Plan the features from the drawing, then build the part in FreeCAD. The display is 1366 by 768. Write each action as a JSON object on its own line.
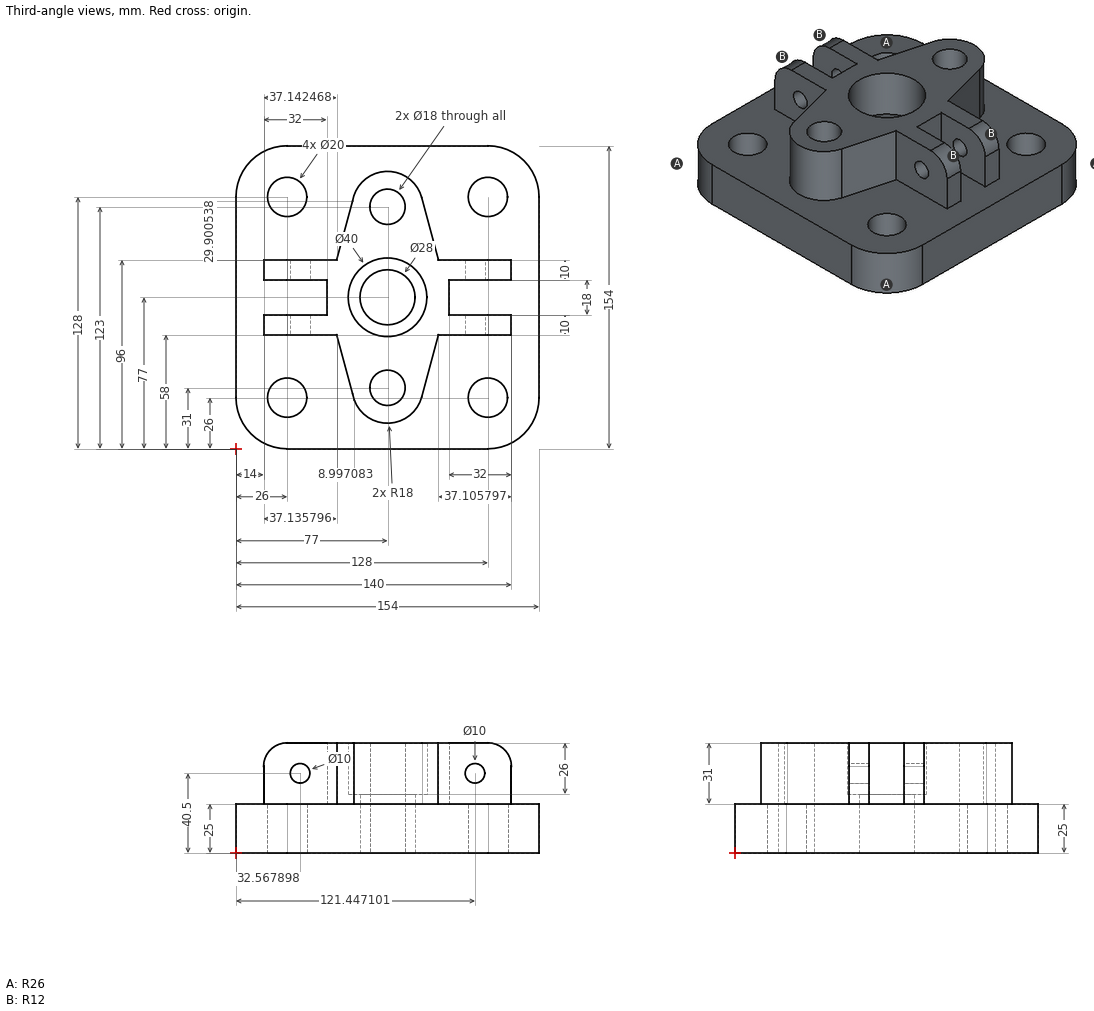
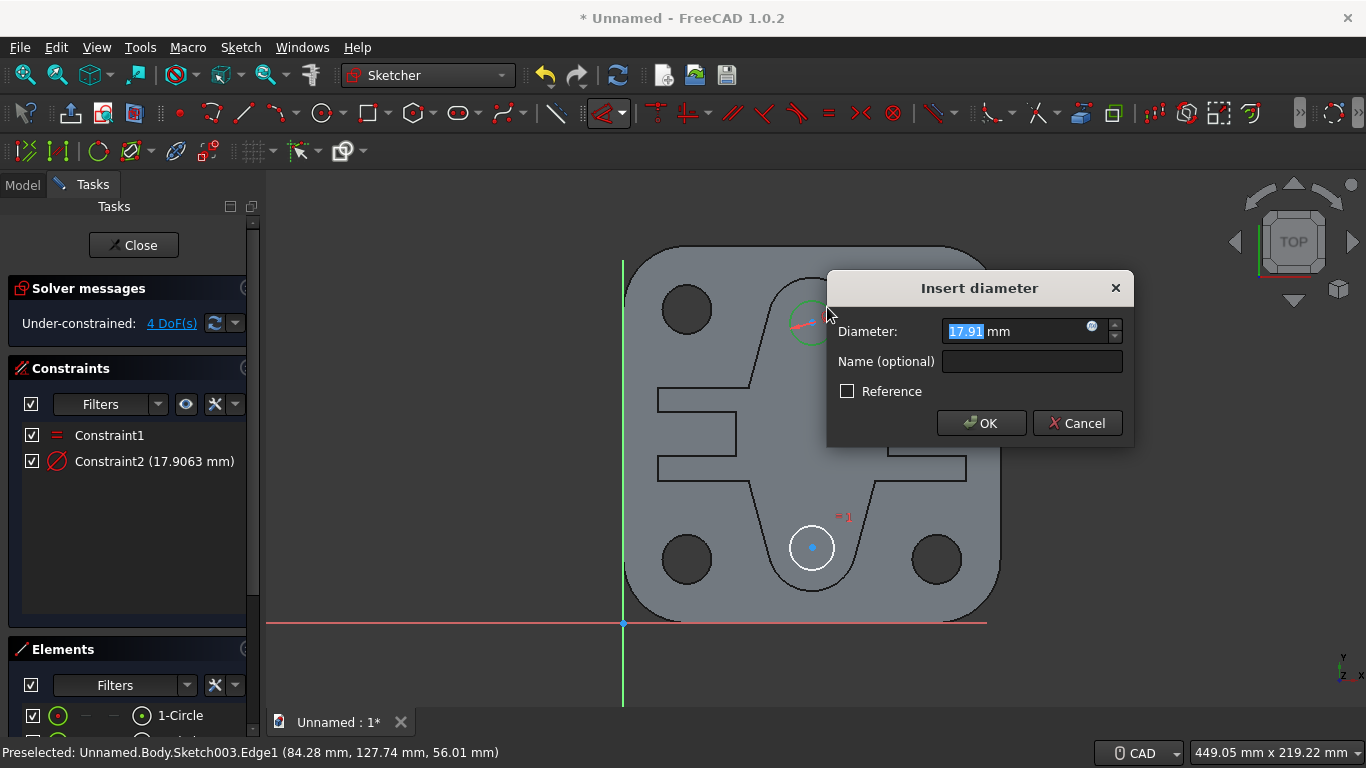
{"action": "type", "text": "18"}
{"action": "key", "text": "Return"}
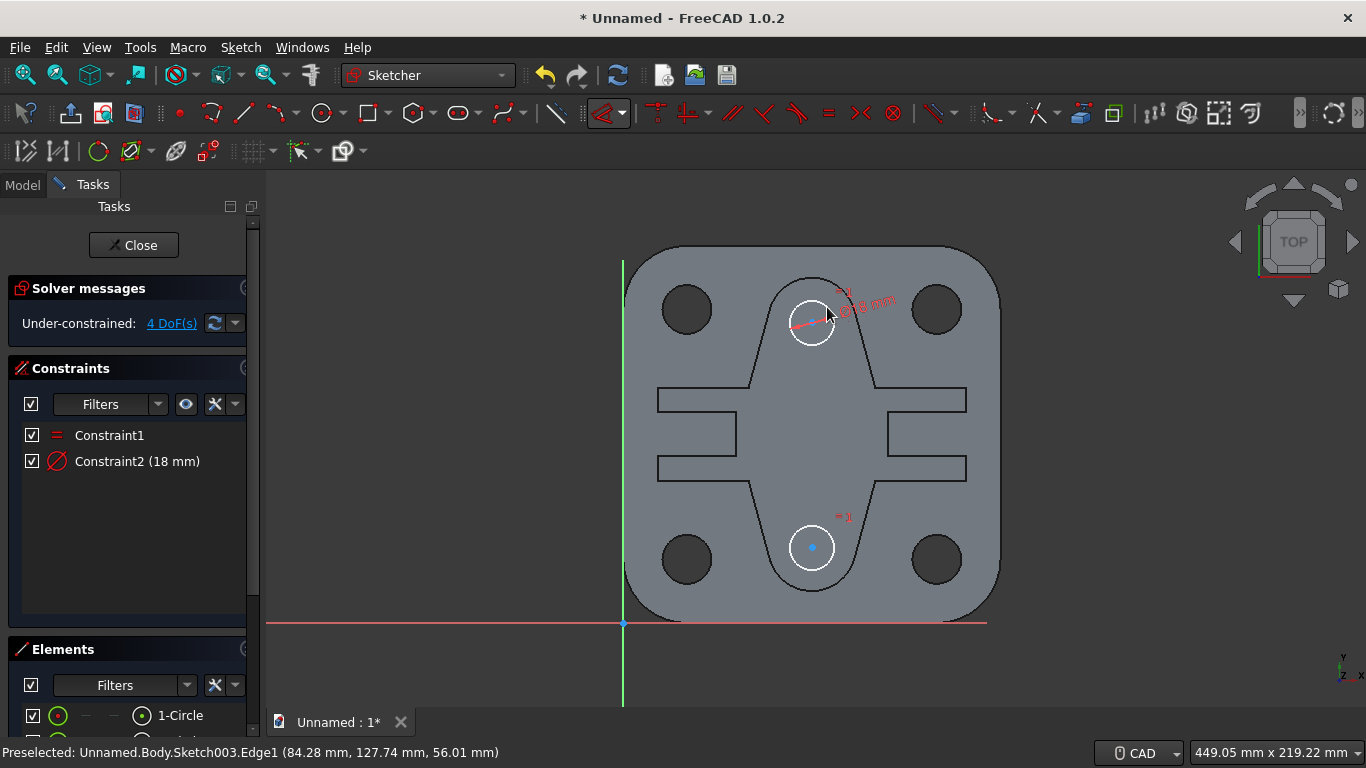
{"action": "left_click", "coordinate": [812, 323]}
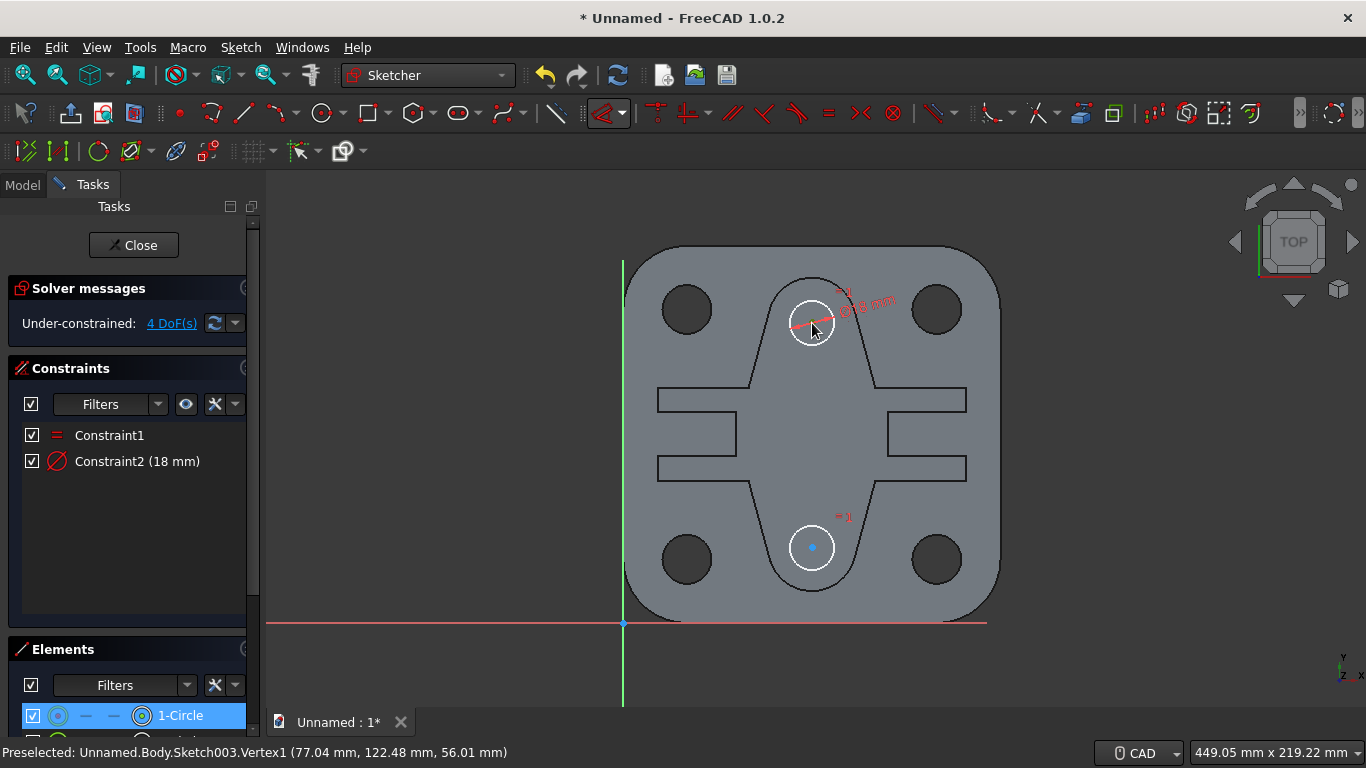
{"action": "key", "text": "l"}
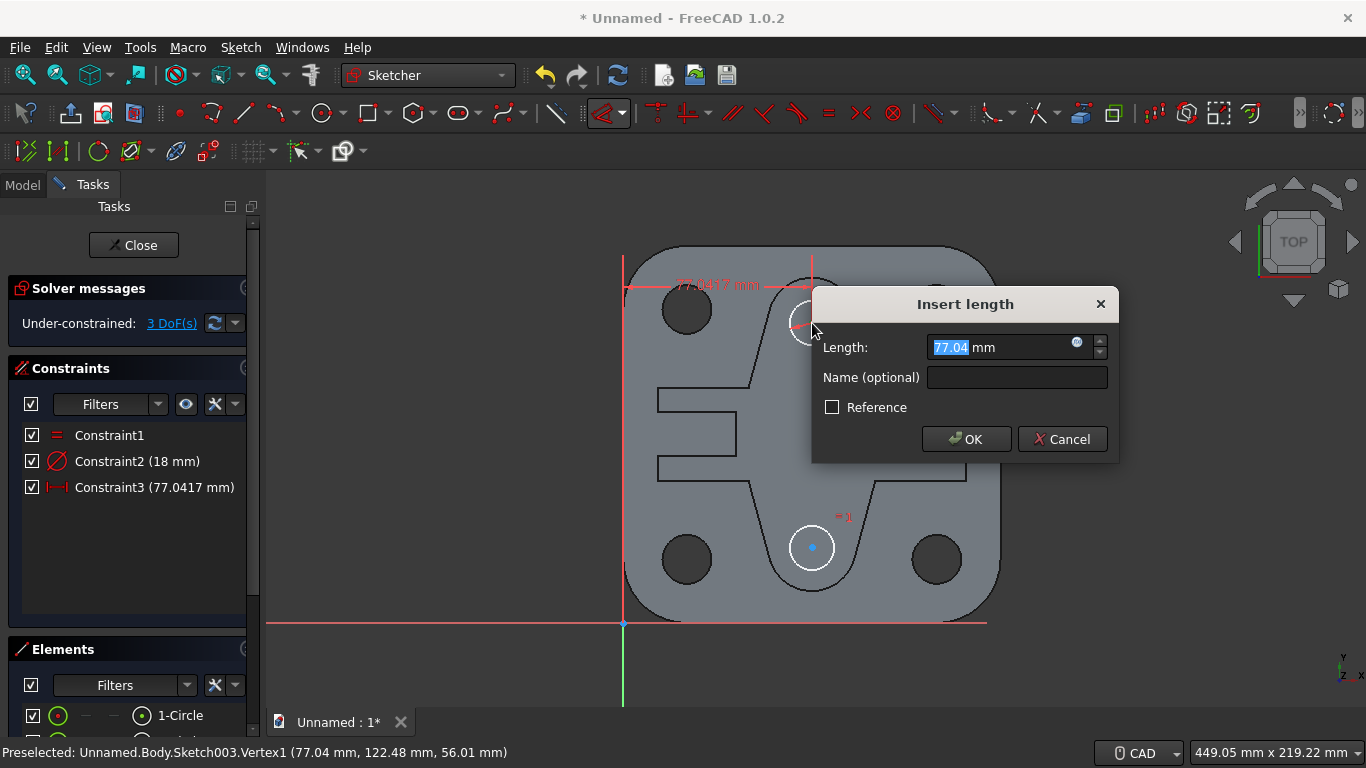
{"action": "type", "text": "77"}
{"action": "key", "text": "Return"}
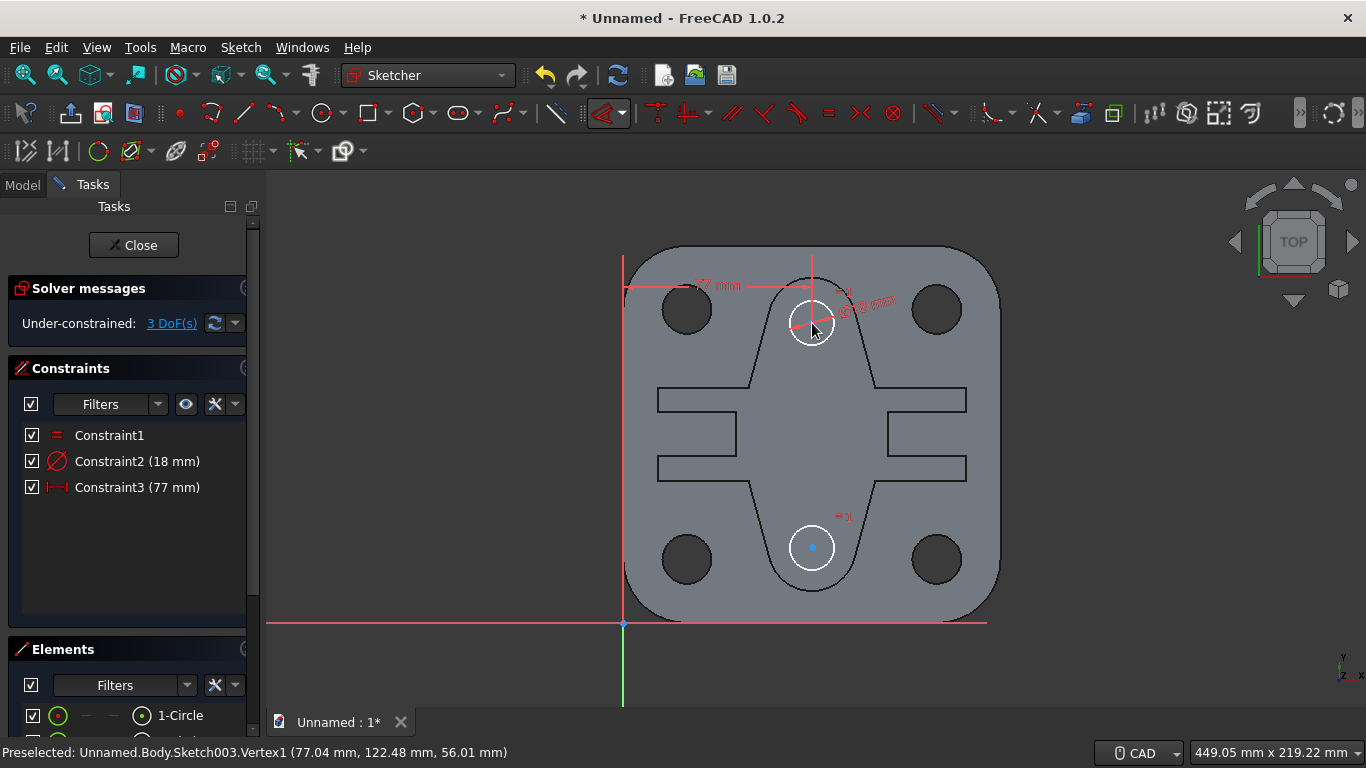
{"action": "left_click", "coordinate": [812, 548]}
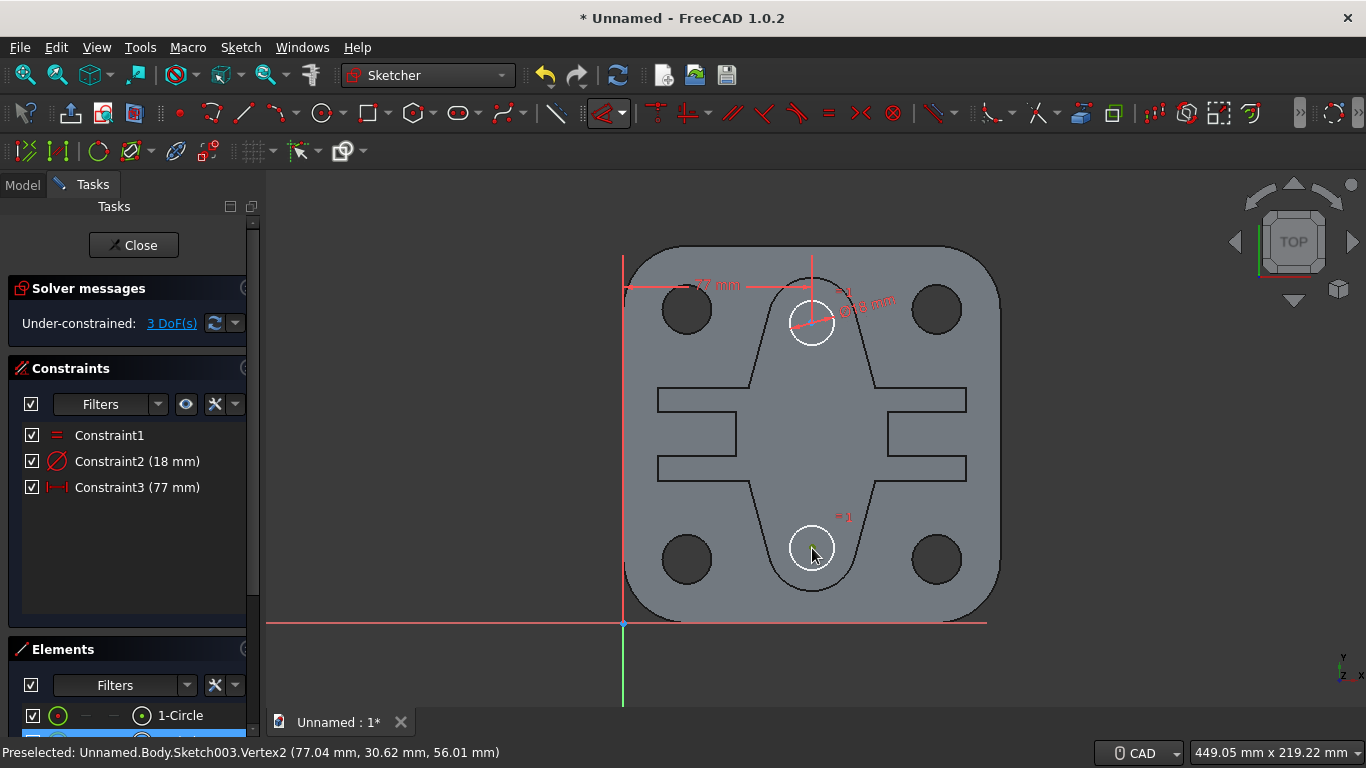
{"action": "left_click", "coordinate": [624, 114]}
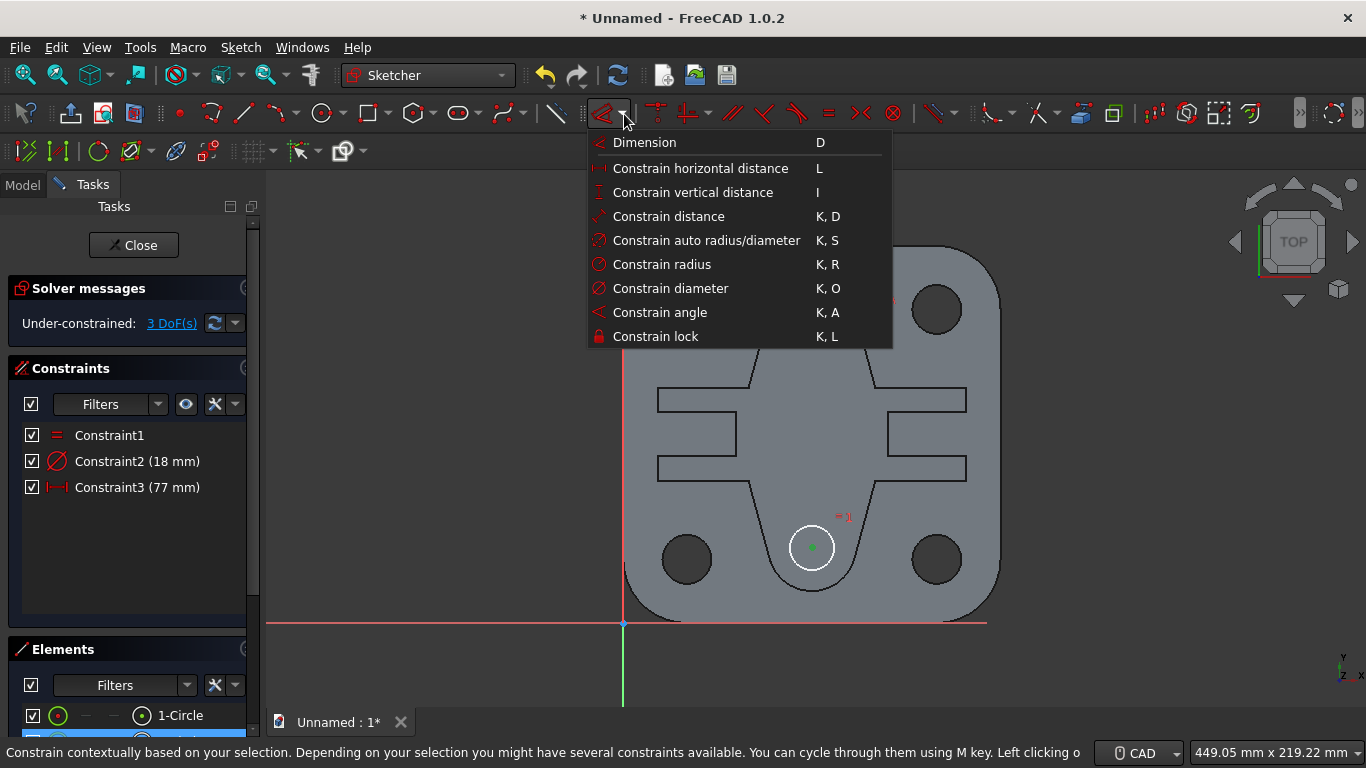
{"action": "left_click", "coordinate": [740, 168]}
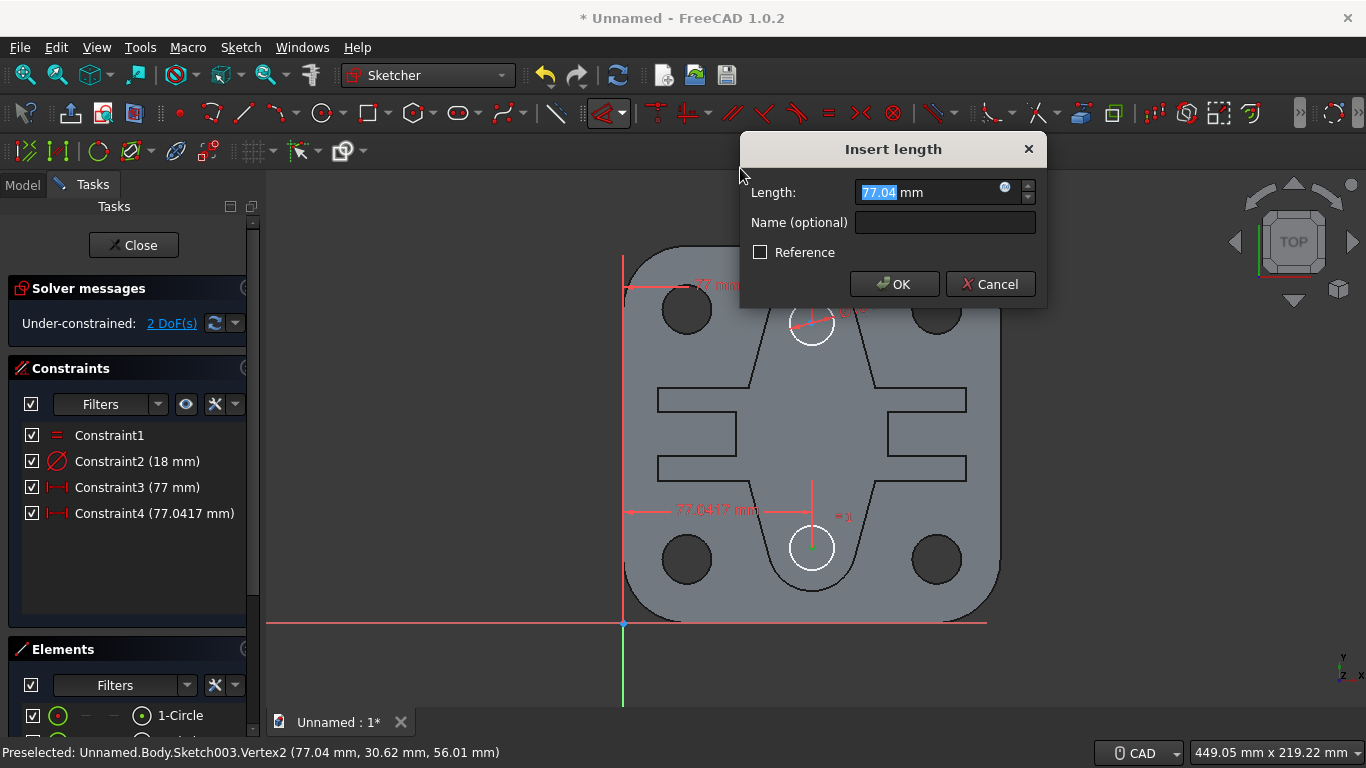
{"action": "type", "text": "77"}
{"action": "key", "text": "Return"}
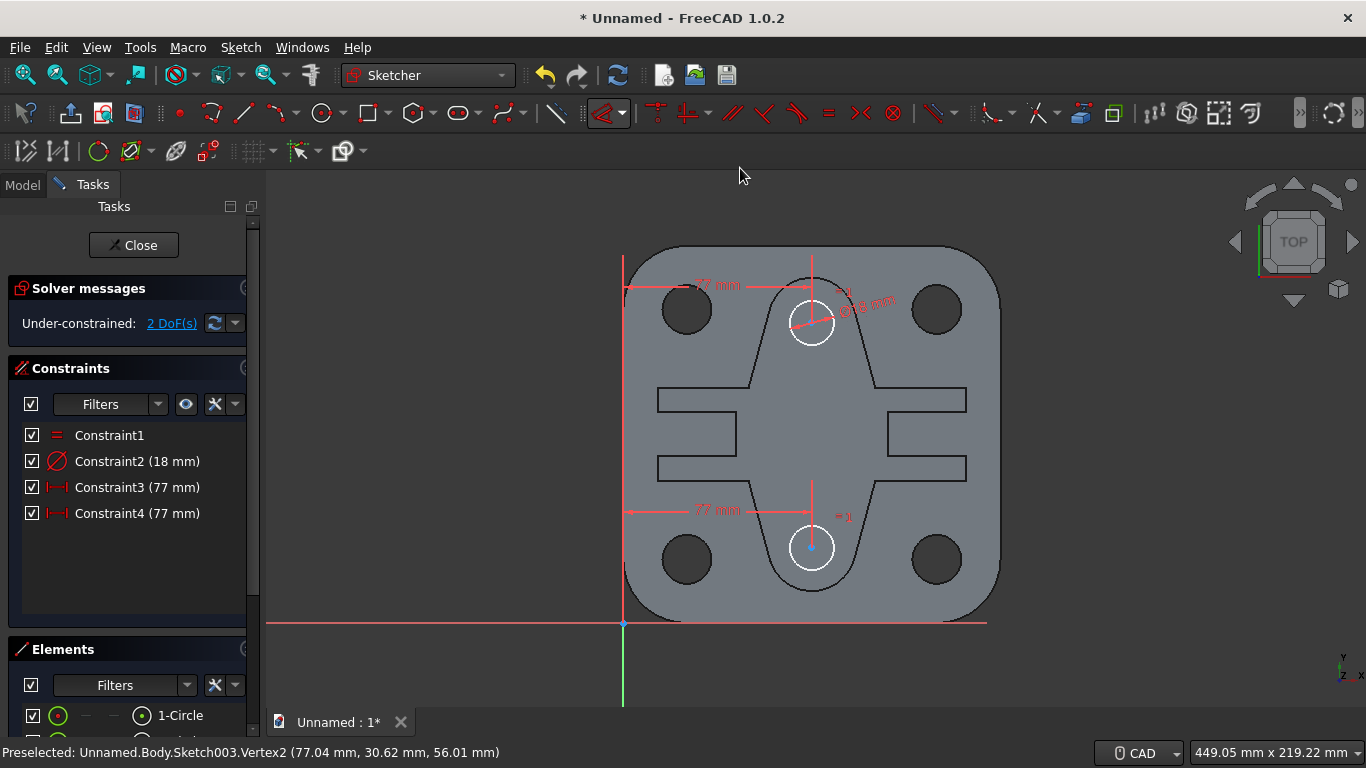
{"action": "left_click", "coordinate": [812, 548]}